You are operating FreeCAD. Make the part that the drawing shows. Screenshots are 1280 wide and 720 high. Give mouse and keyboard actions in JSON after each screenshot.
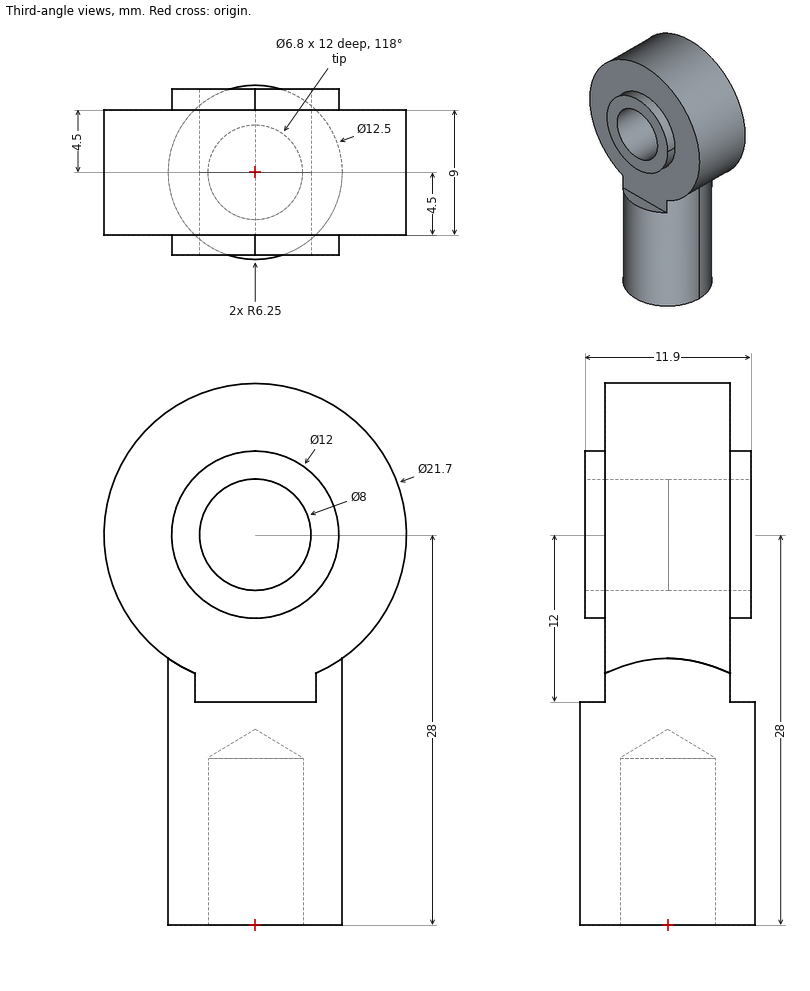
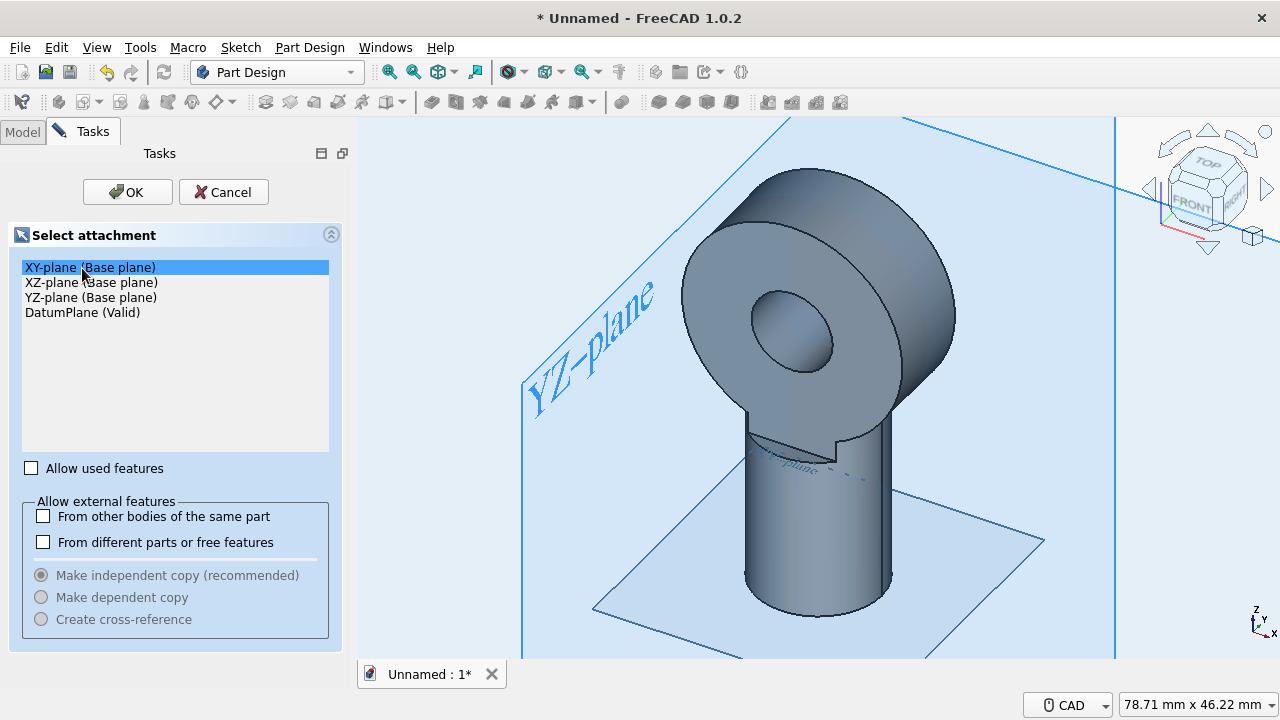
{"action": "left_click", "coordinate": [128, 192]}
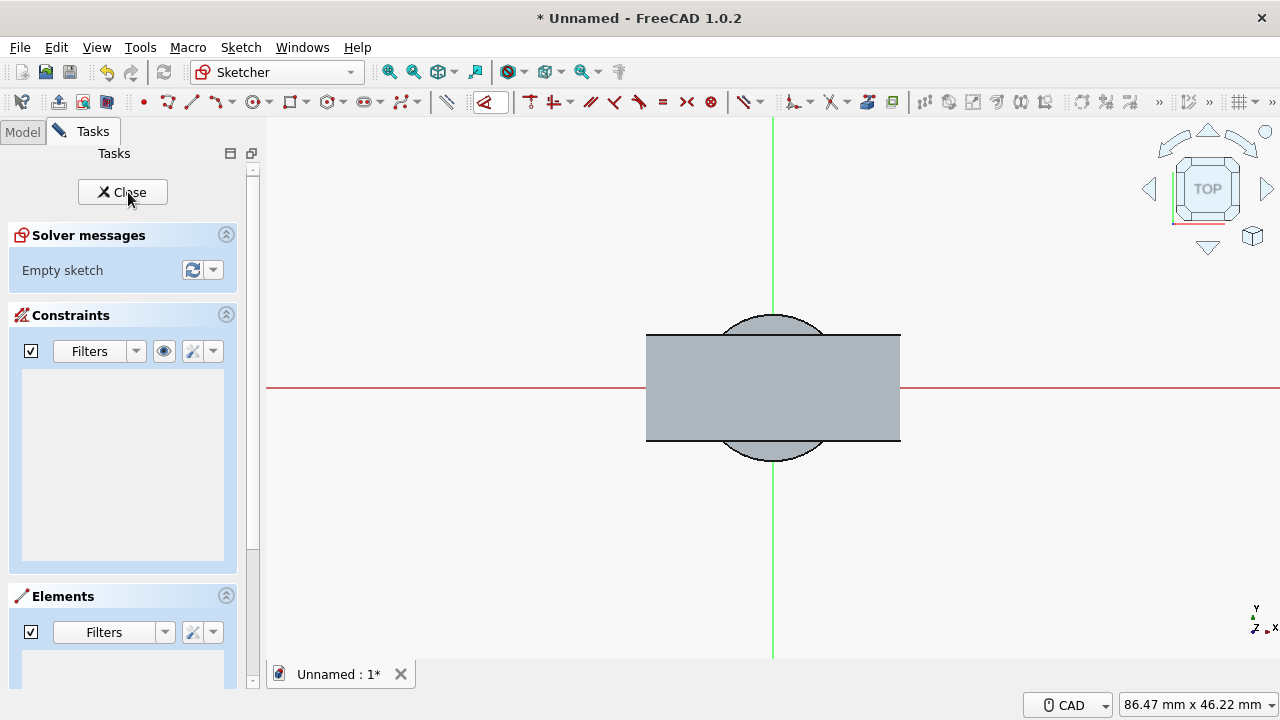
{"action": "left_click", "coordinate": [108, 102]}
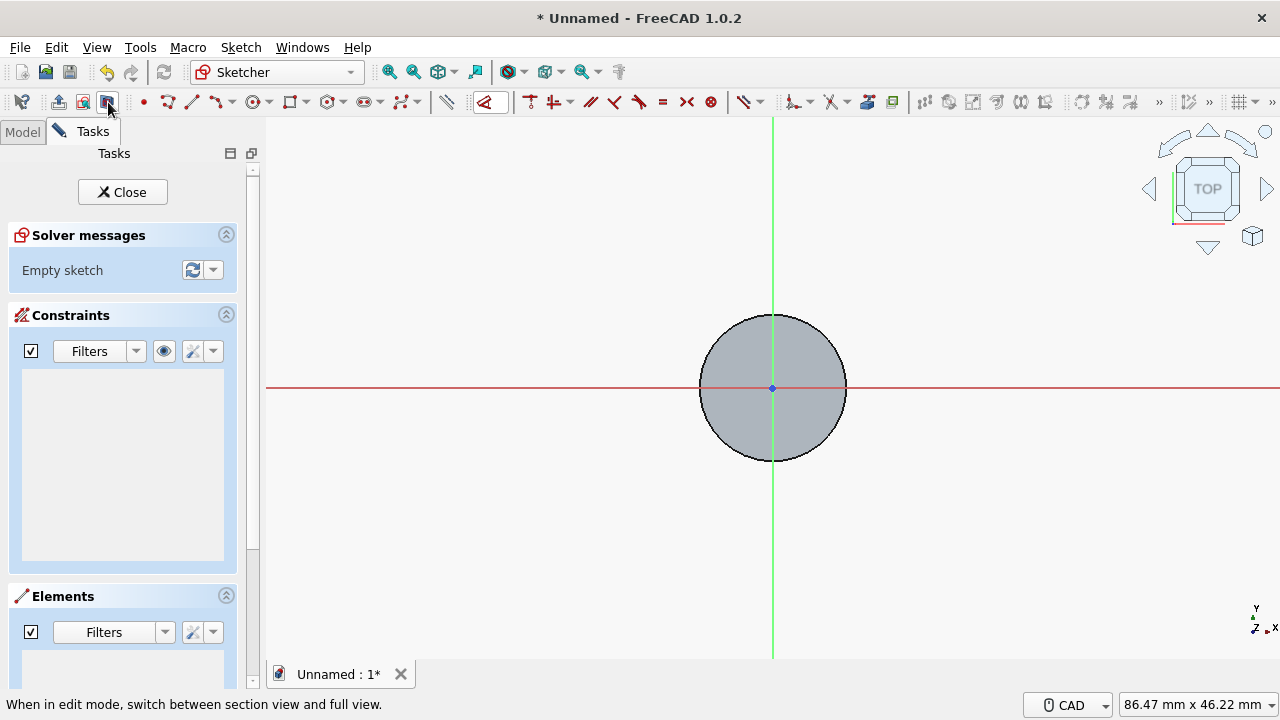
{"action": "scroll", "coordinate": [795, 388], "scroll_direction": "up", "scroll_amount": 7}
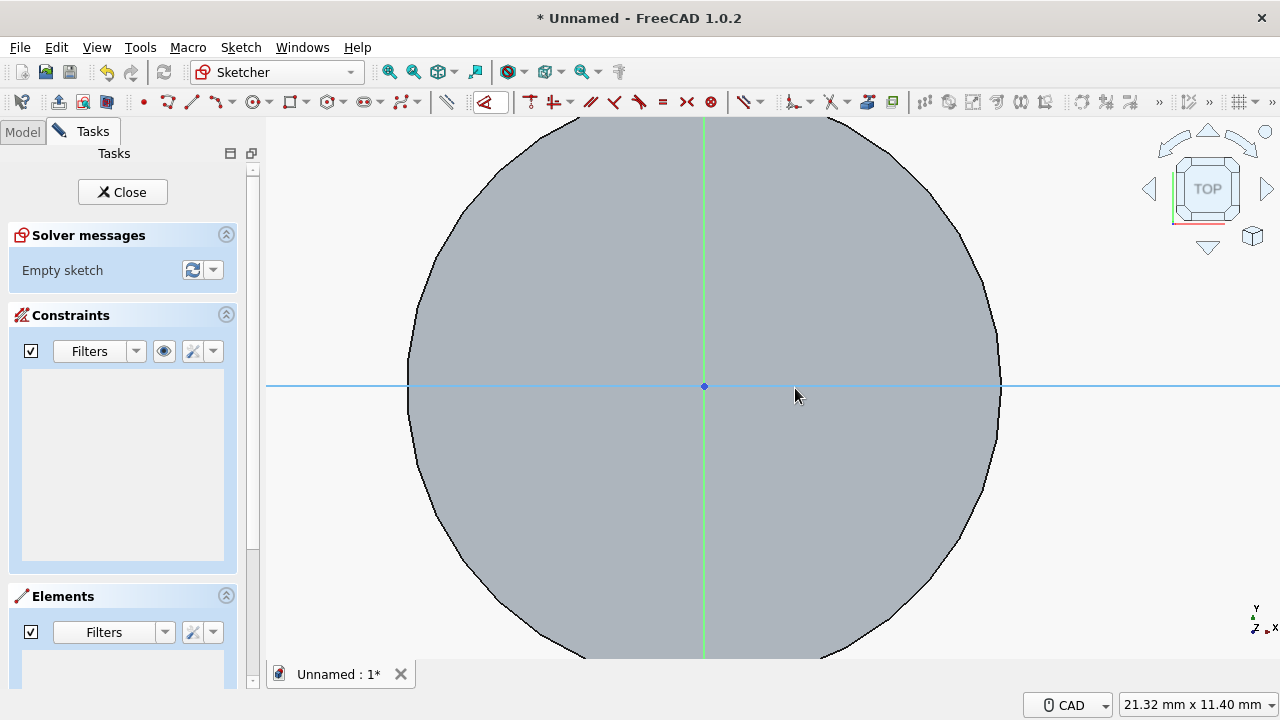
{"action": "left_click", "coordinate": [254, 102]}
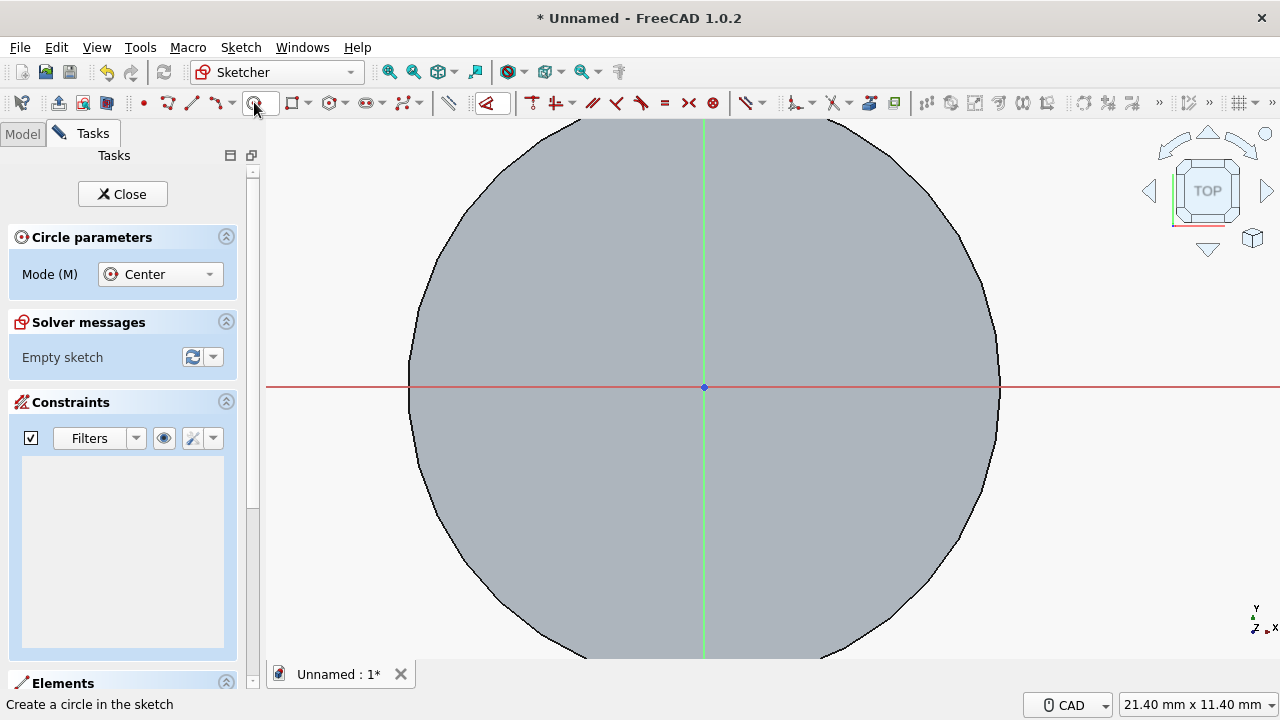
{"action": "left_click", "coordinate": [704, 387]}
{"action": "left_click", "coordinate": [818, 274]}
{"action": "key", "text": "Escape"}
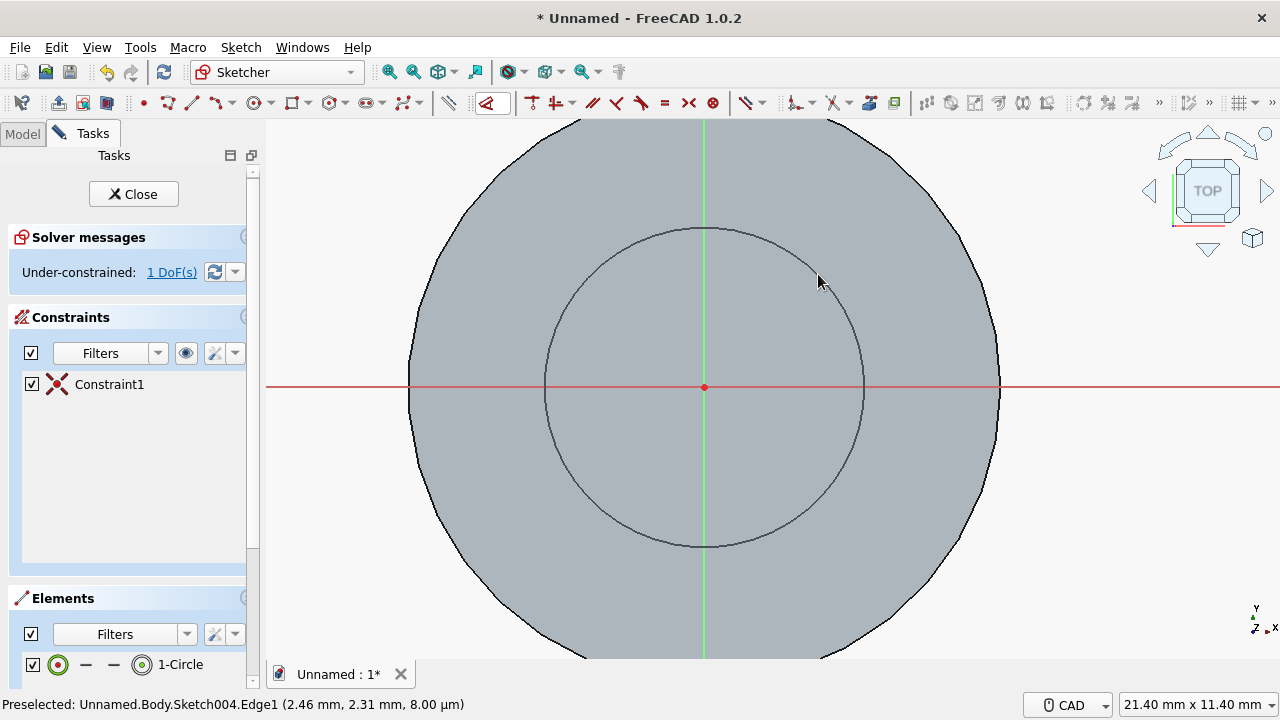
{"action": "left_click", "coordinate": [817, 274]}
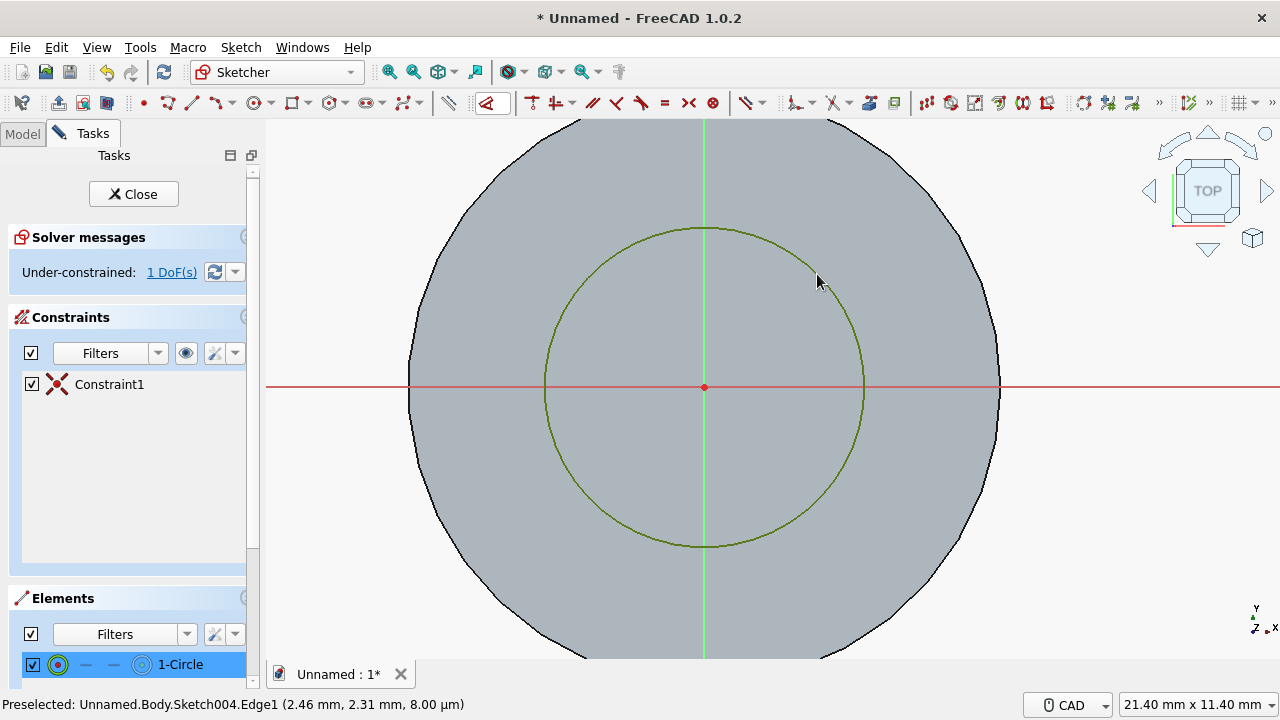
{"action": "key", "text": "k o"}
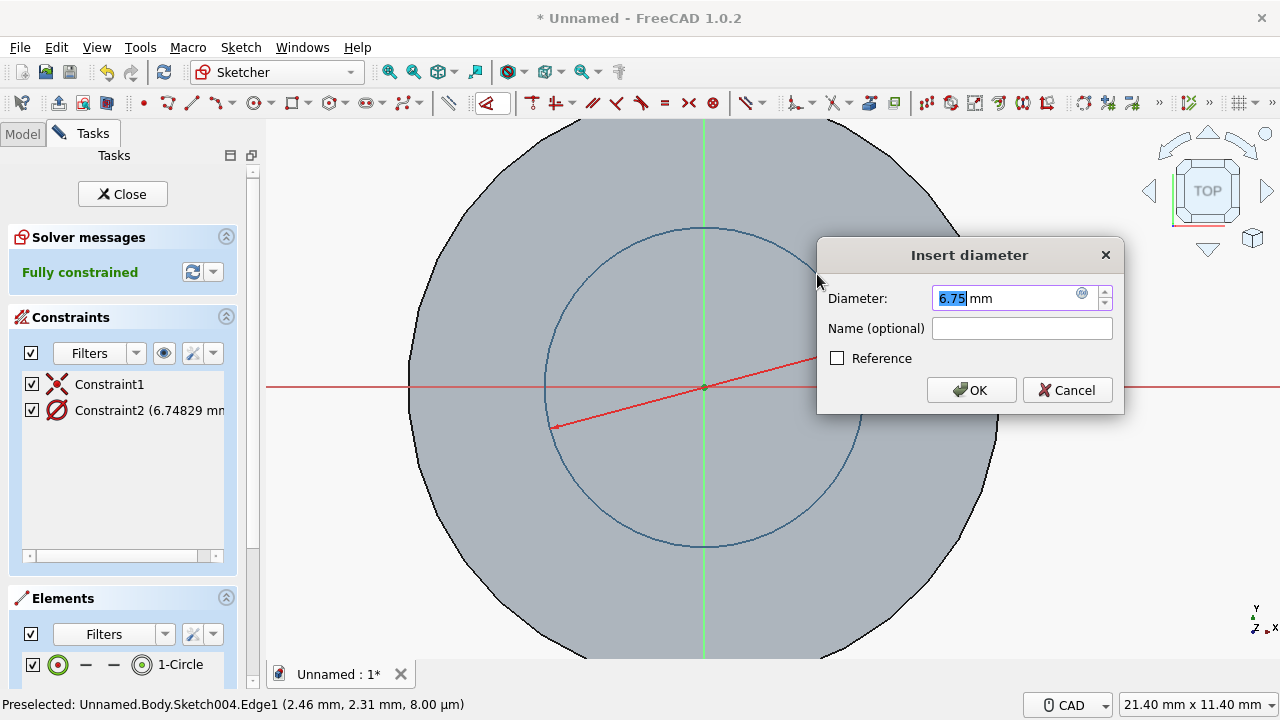
{"action": "type", "text": "6.8"}
{"action": "key", "text": "Return"}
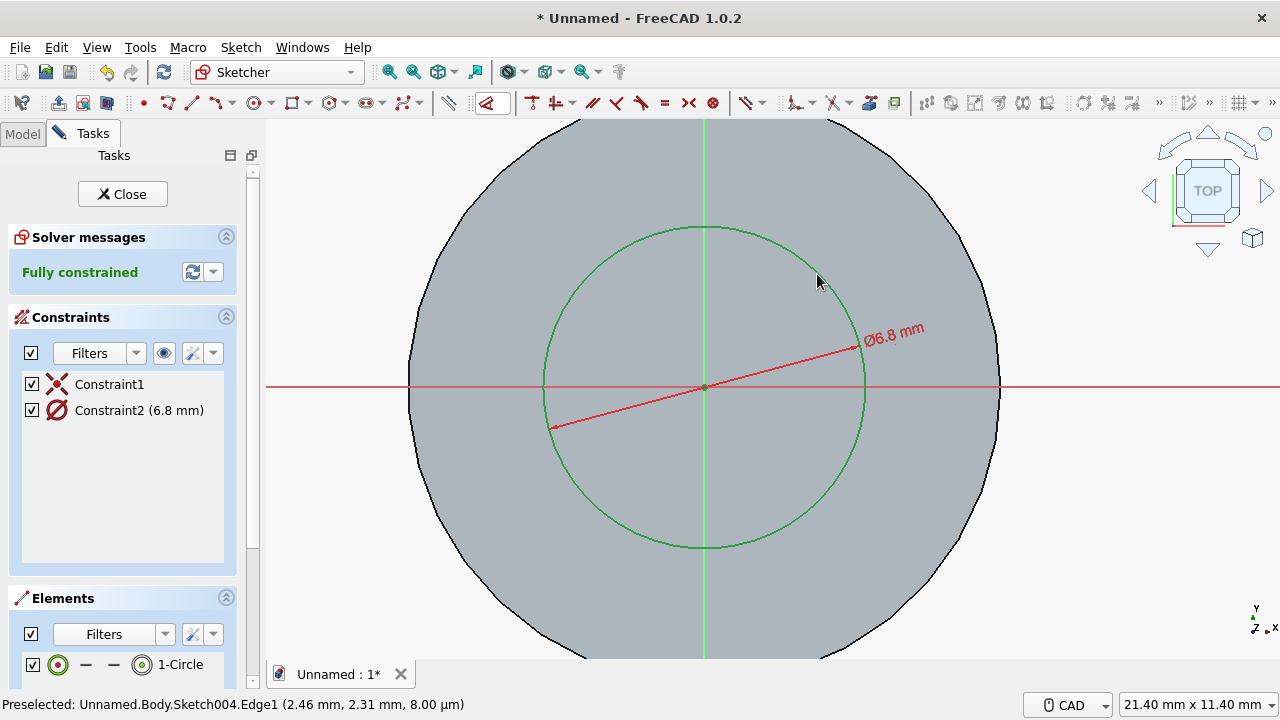
{"action": "left_click", "coordinate": [123, 194]}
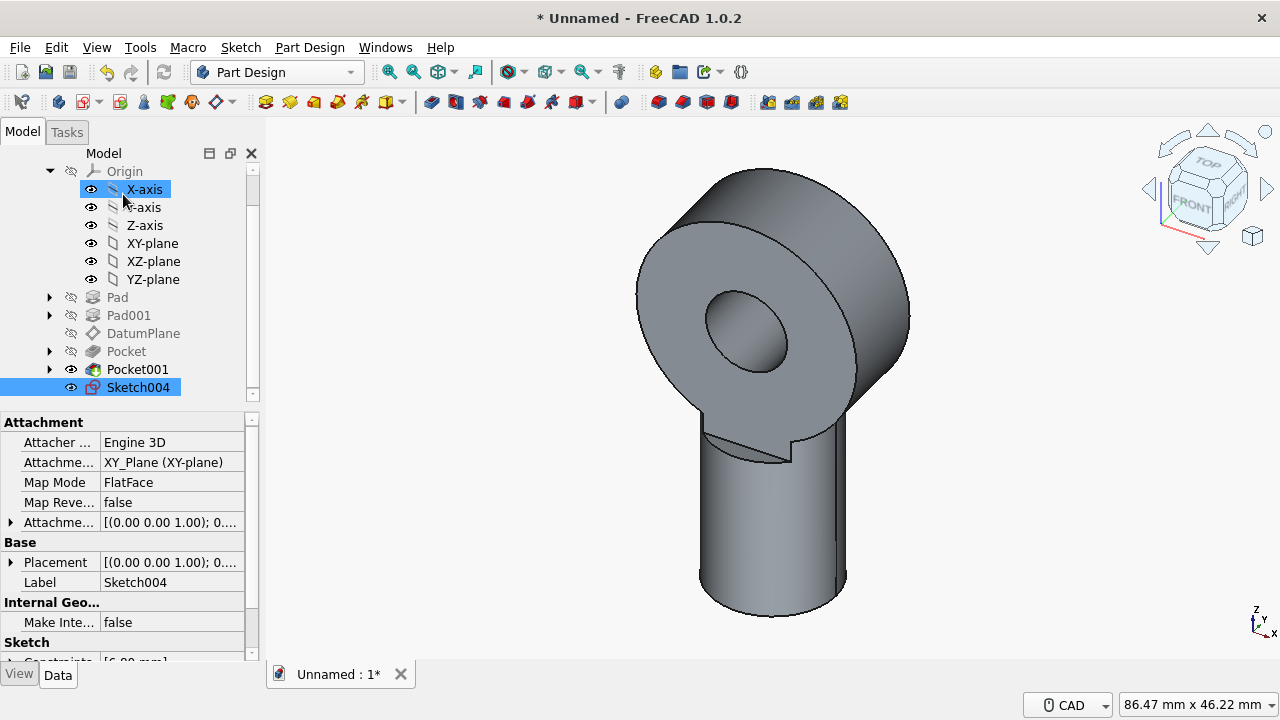
{"action": "left_click", "coordinate": [456, 102]}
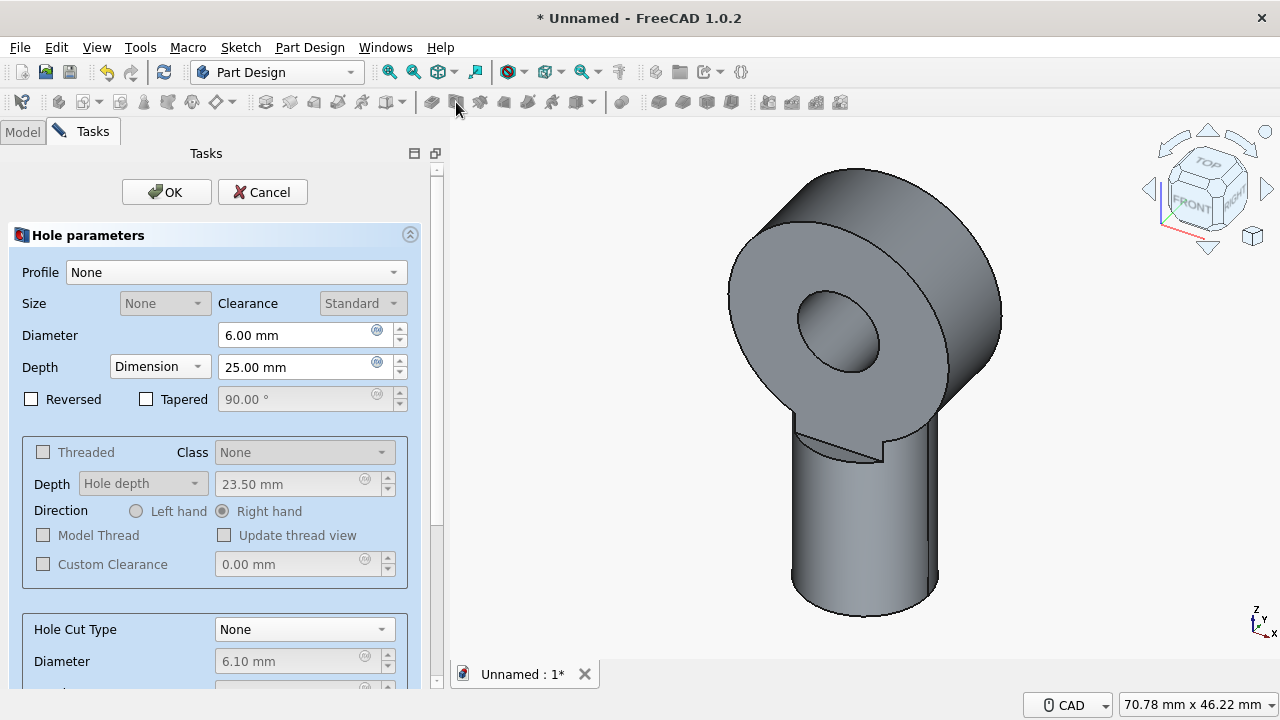
{"action": "triple_click", "coordinate": [305, 335]}